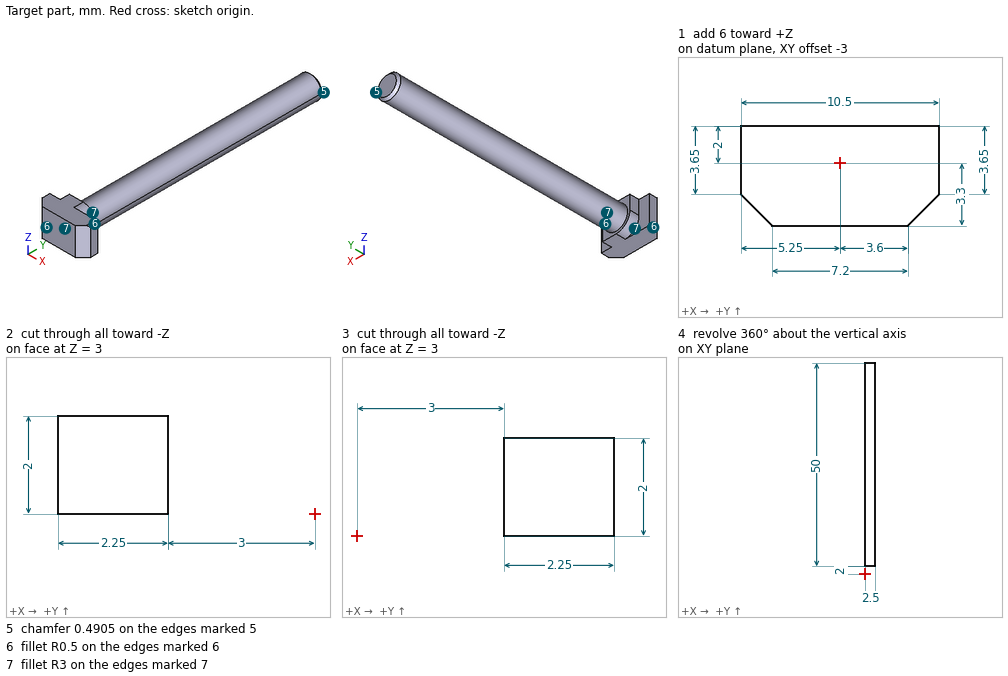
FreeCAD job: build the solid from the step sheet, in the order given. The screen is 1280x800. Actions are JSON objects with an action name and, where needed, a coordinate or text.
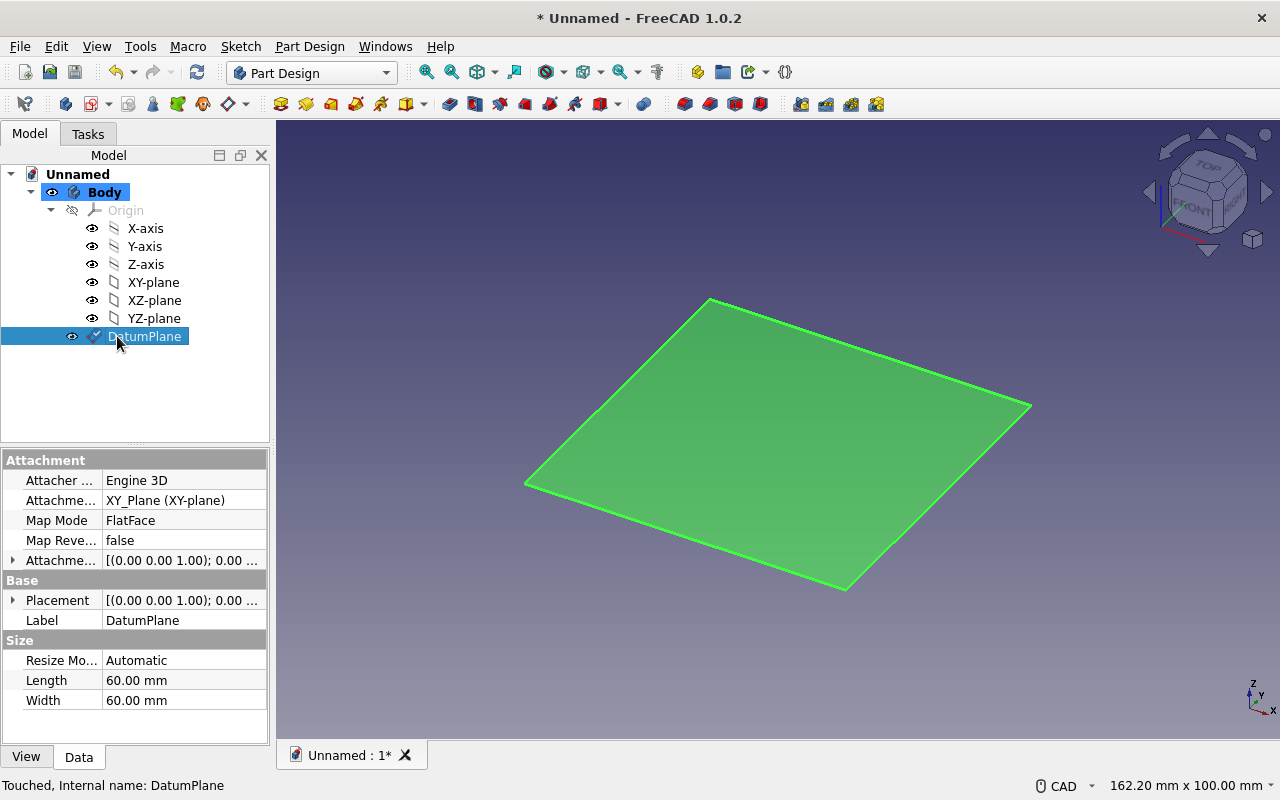
{"action": "left_click", "coordinate": [90, 104]}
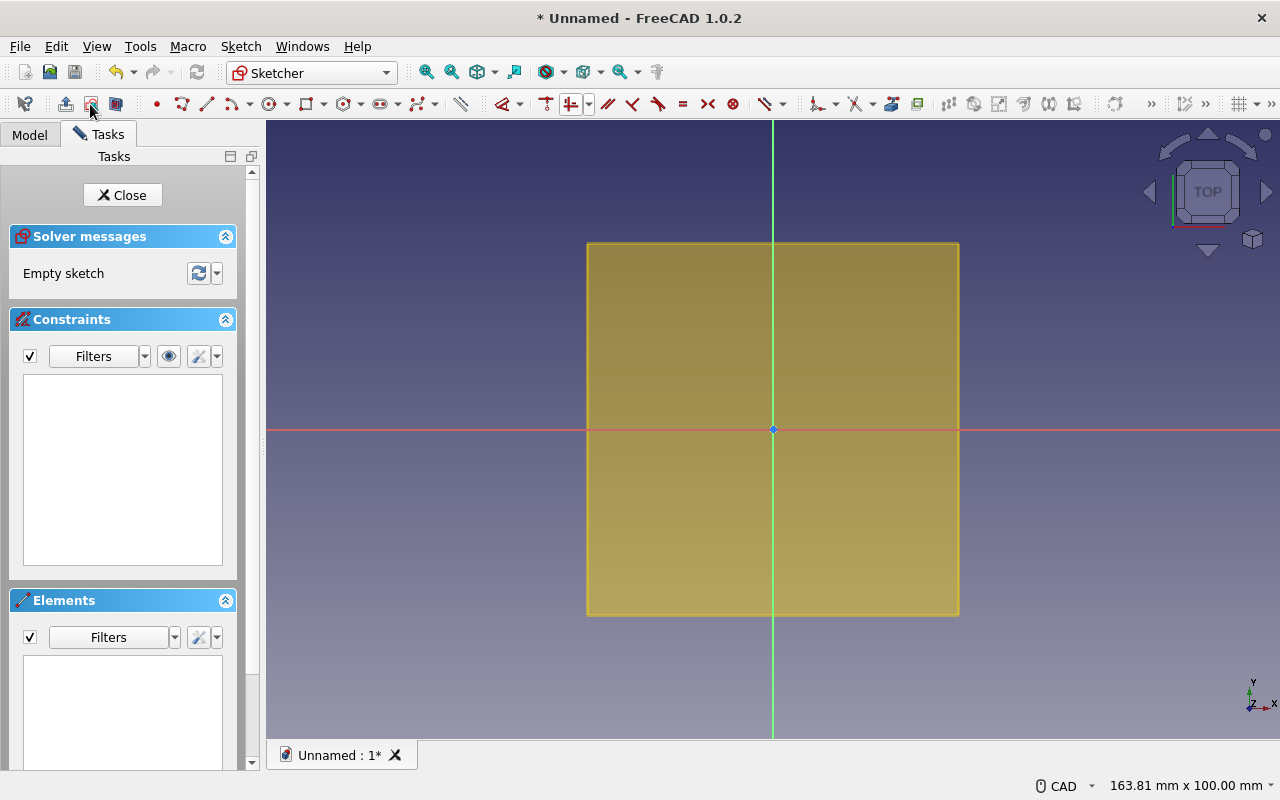
{"action": "scroll", "coordinate": [782, 434], "scroll_direction": "up", "scroll_amount": 11}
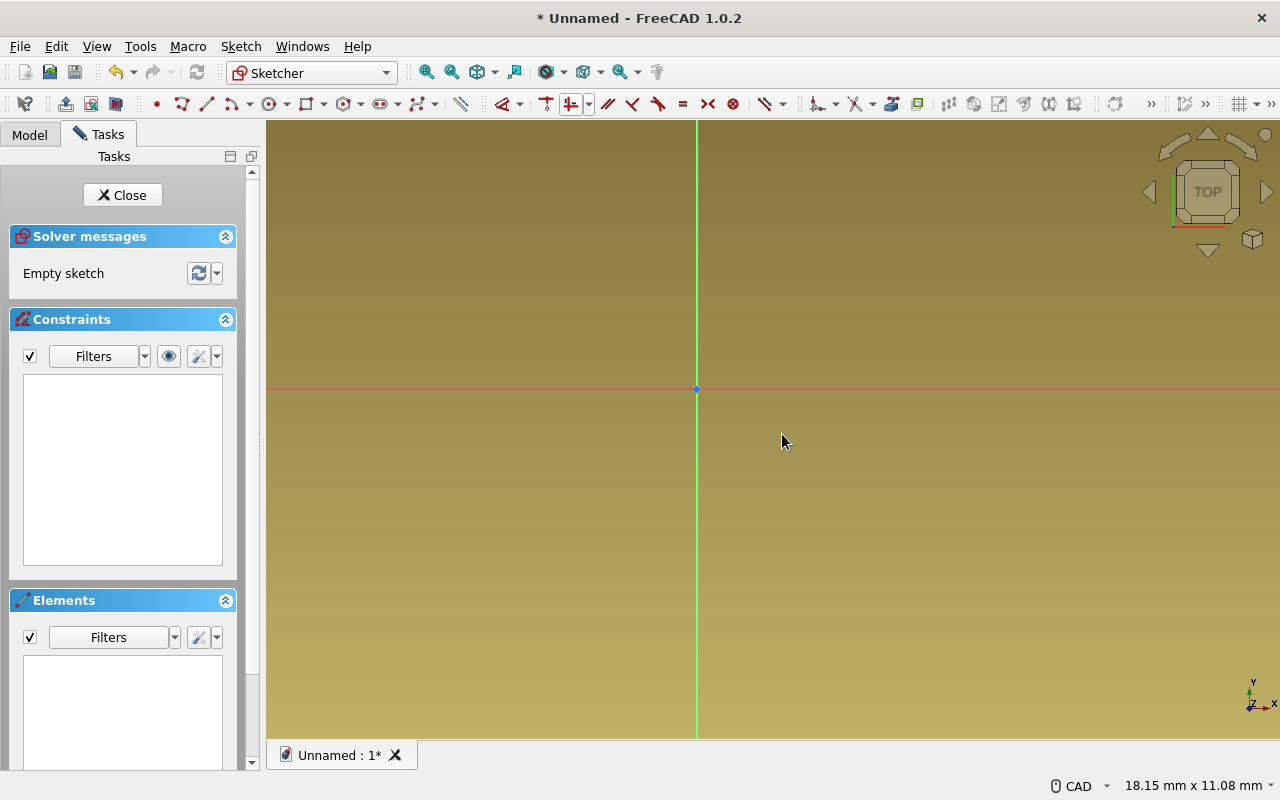
{"action": "left_click", "coordinate": [182, 104]}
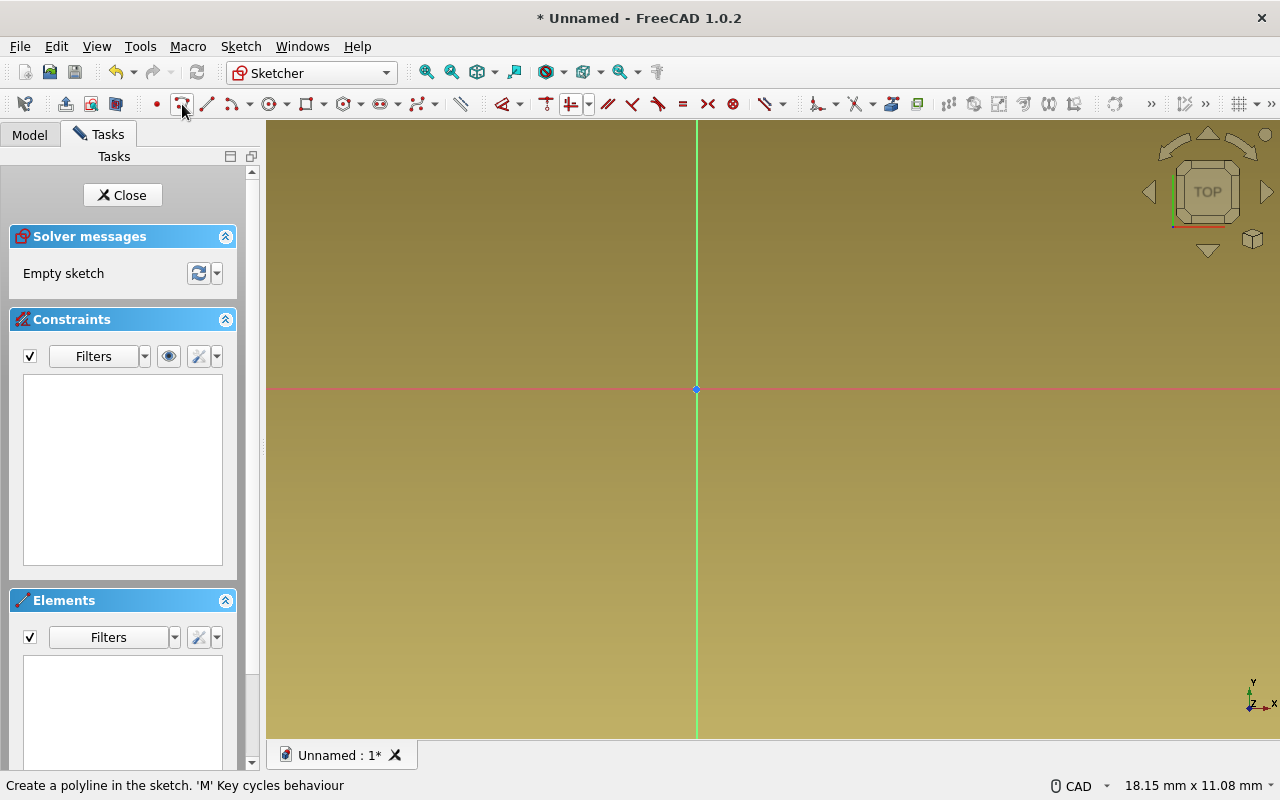
{"action": "left_click", "coordinate": [898, 574]}
{"action": "left_click", "coordinate": [496, 574]}
{"action": "left_click", "coordinate": [403, 481]}
{"action": "left_click", "coordinate": [403, 278]}
{"action": "left_click", "coordinate": [990, 278]}
{"action": "left_click", "coordinate": [990, 481]}
{"action": "left_click", "coordinate": [898, 575]}
{"action": "key", "text": "Escape"}
{"action": "key", "text": "Escape"}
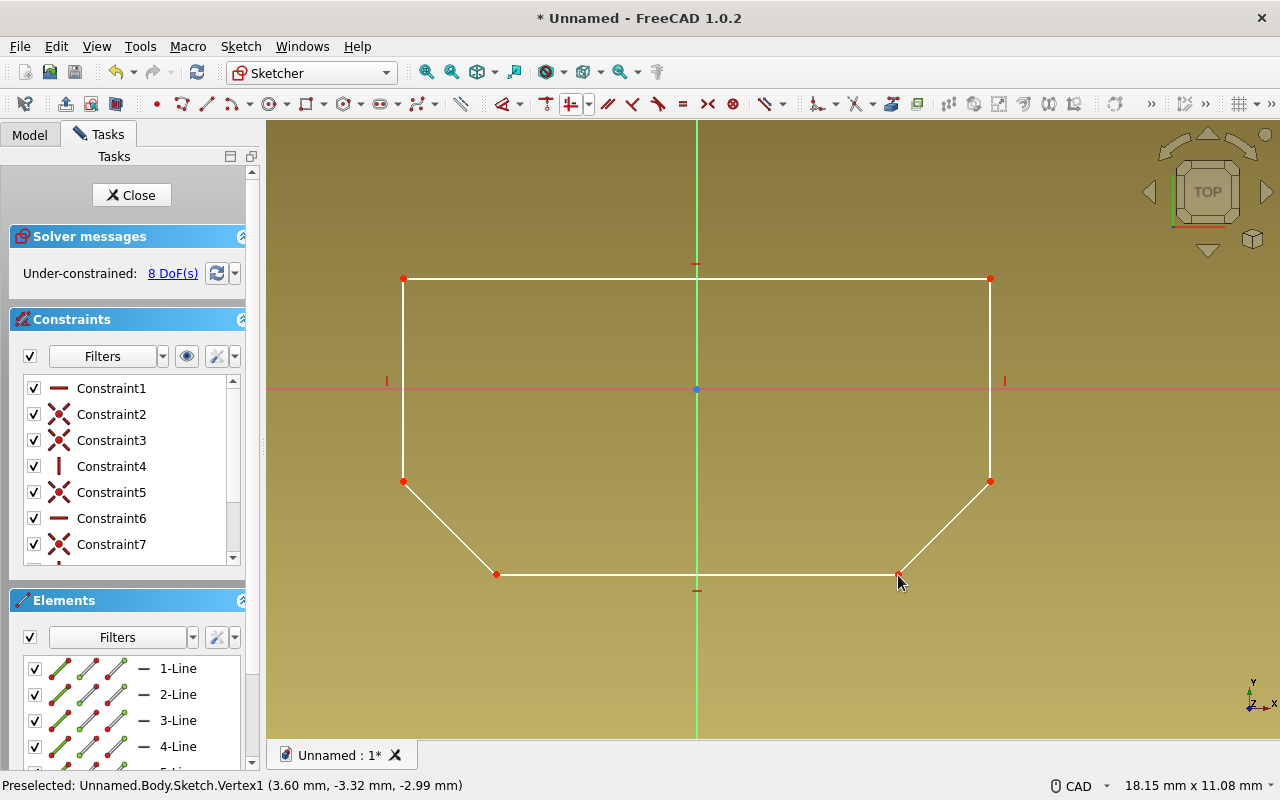
{"action": "left_click", "coordinate": [502, 104]}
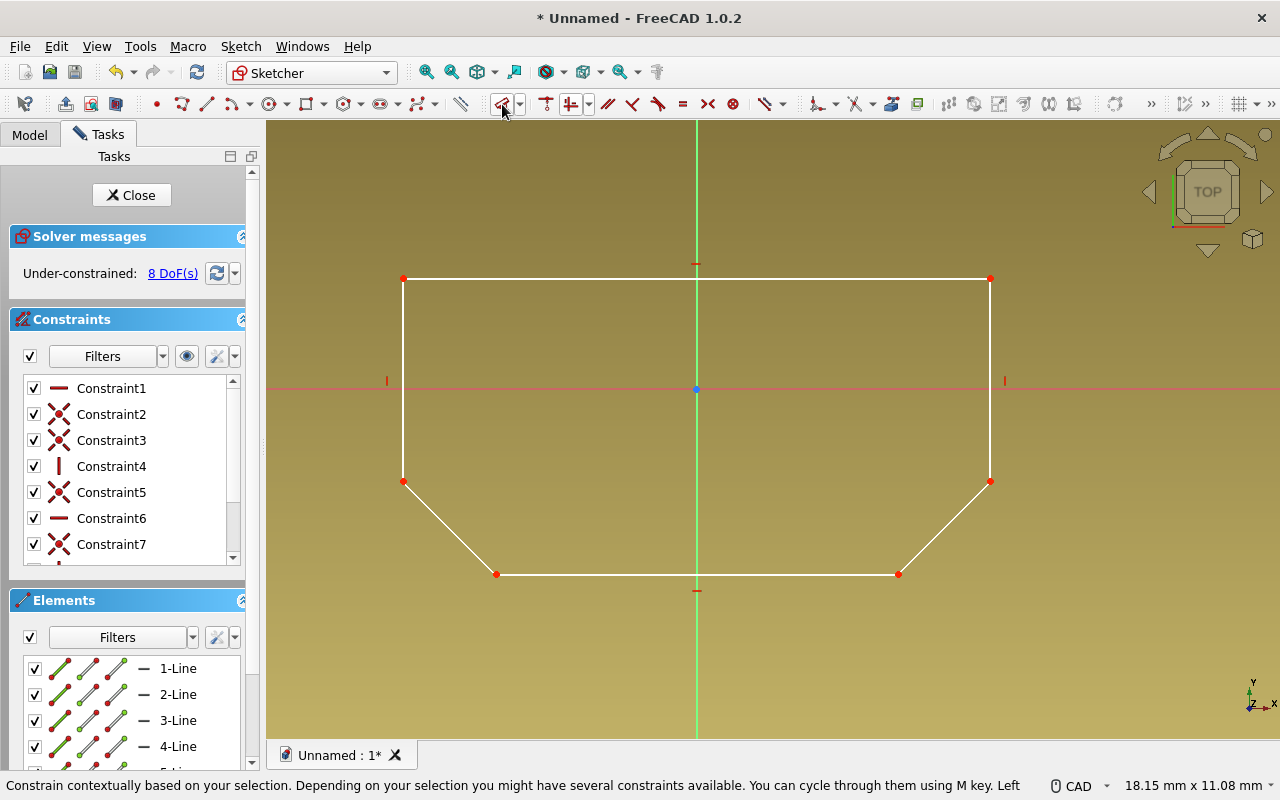
{"action": "left_click", "coordinate": [403, 279]}
{"action": "left_click", "coordinate": [369, 334]}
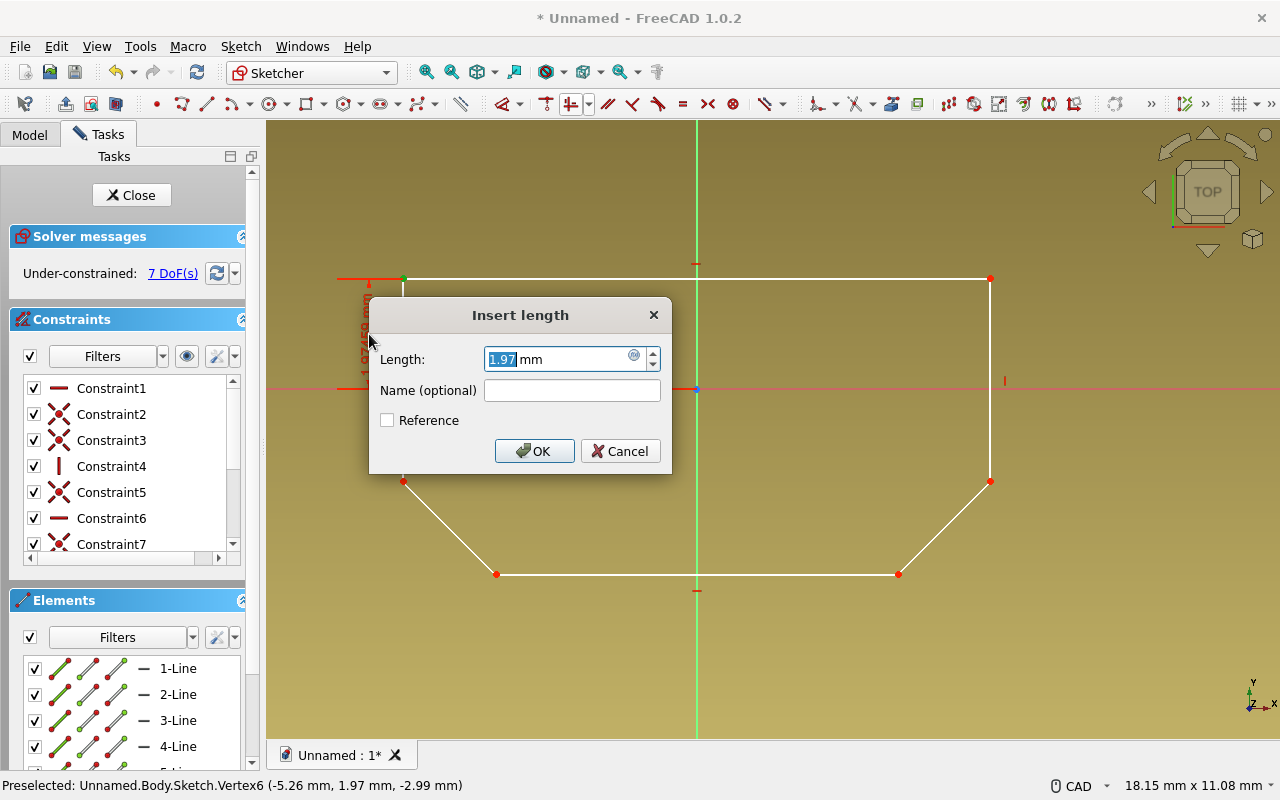
{"action": "type", "text": "2"}
{"action": "key", "text": "Return"}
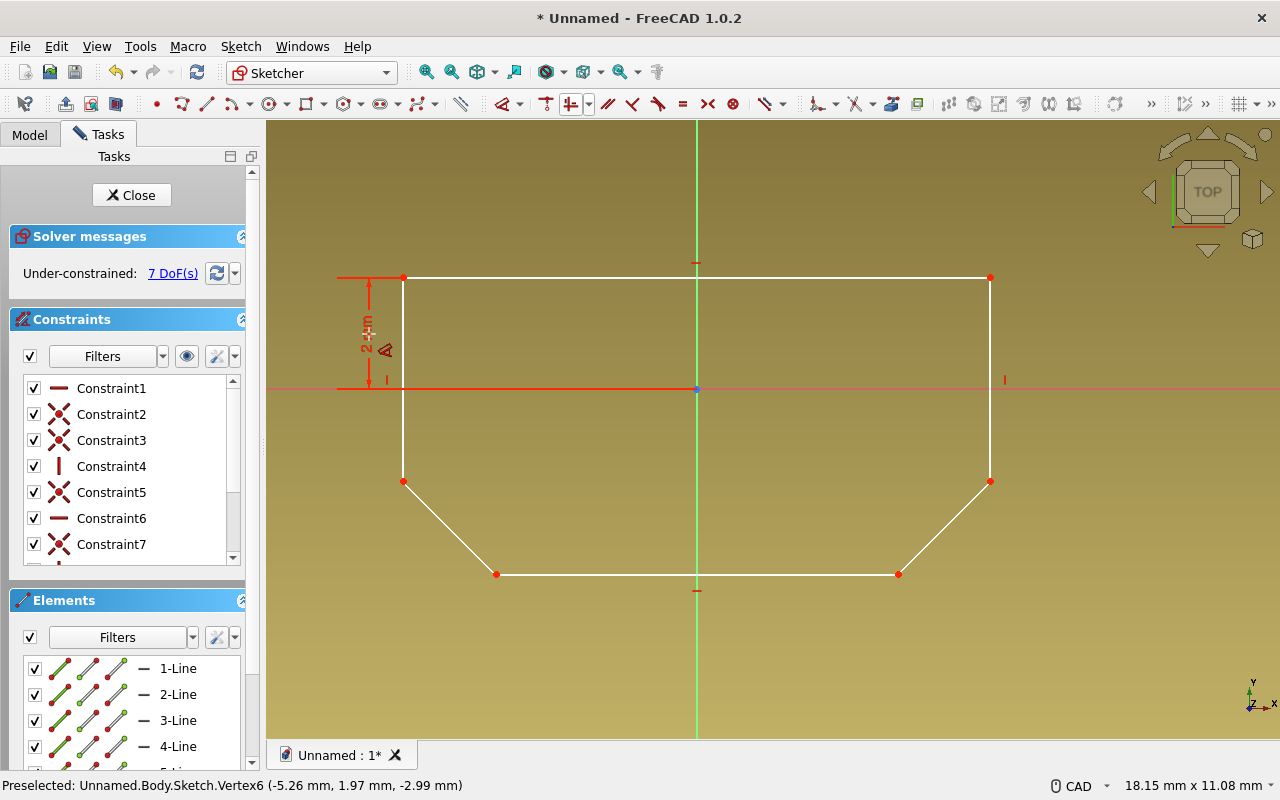
{"action": "left_click", "coordinate": [777, 575]}
{"action": "left_click", "coordinate": [605, 609]}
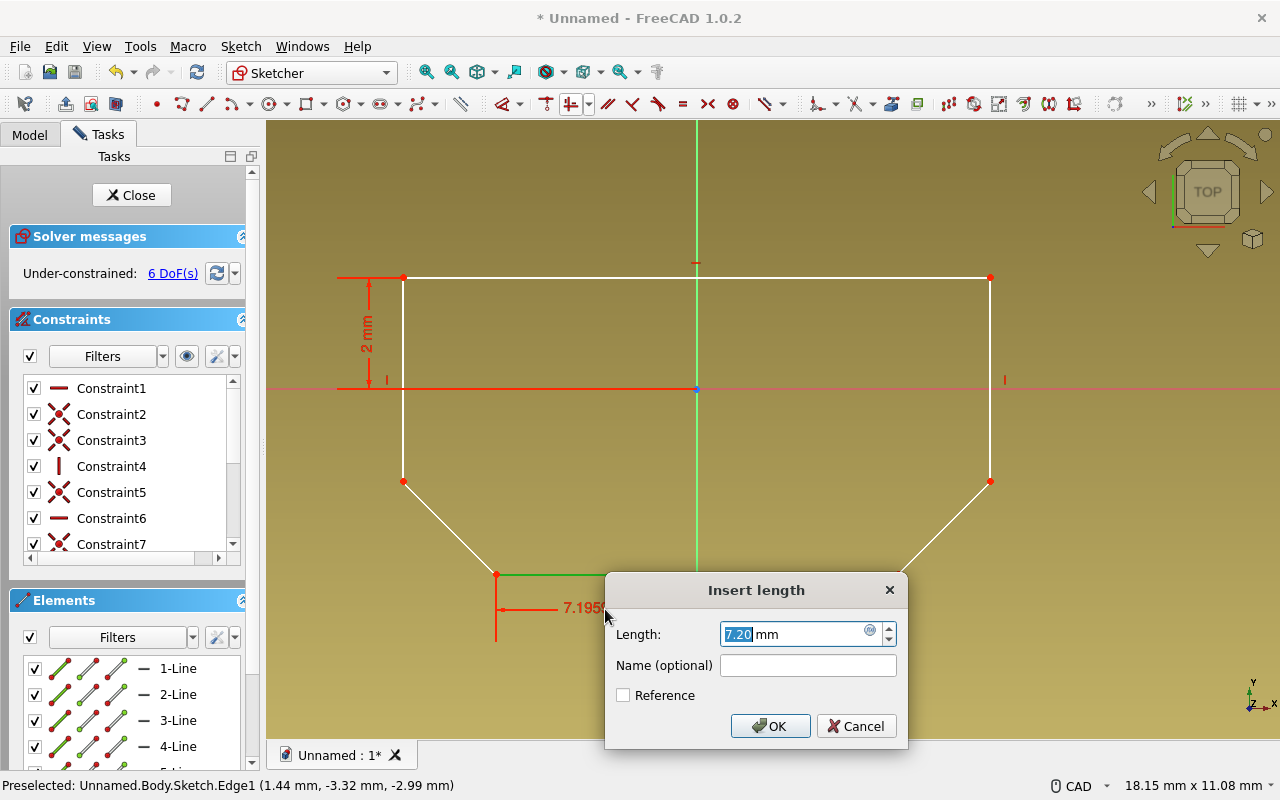
{"action": "type", "text": "7.2"}
{"action": "key", "text": "Return"}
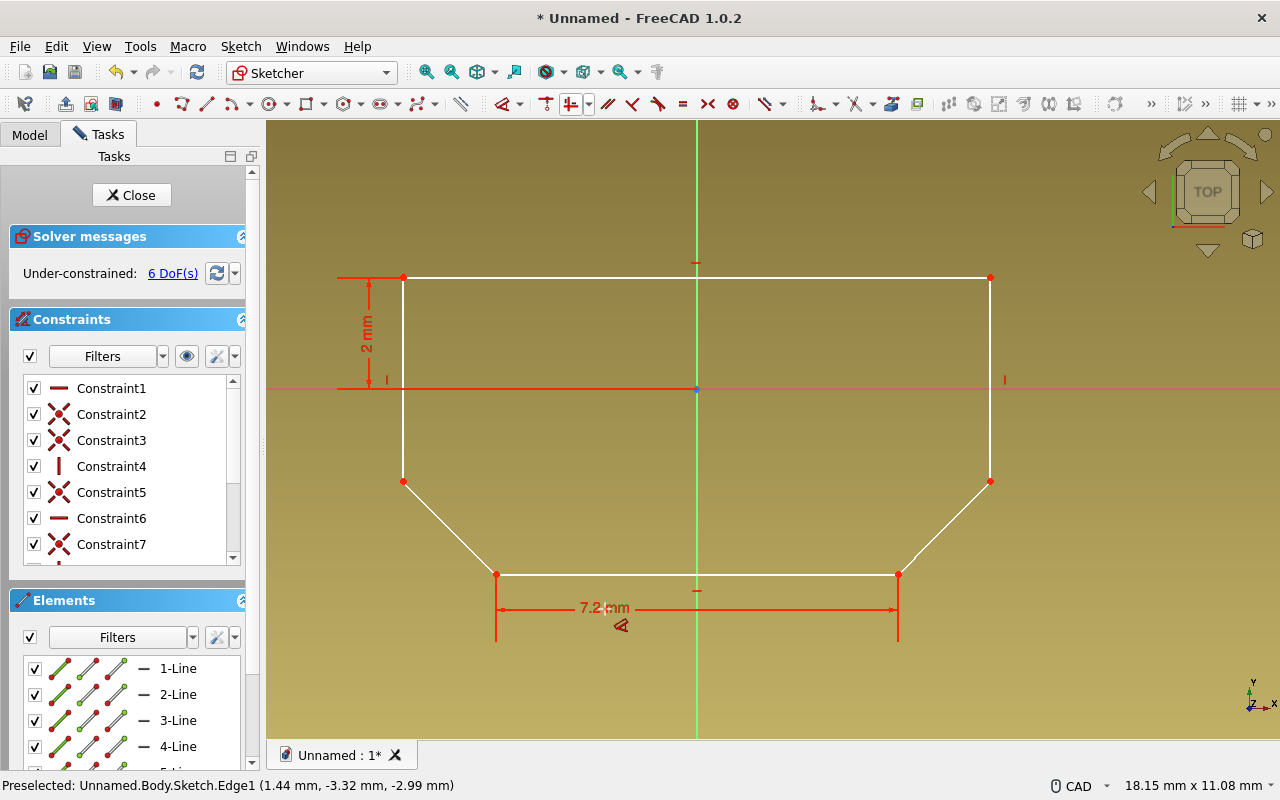
{"action": "left_click", "coordinate": [403, 421]}
{"action": "left_click", "coordinate": [369, 427]}